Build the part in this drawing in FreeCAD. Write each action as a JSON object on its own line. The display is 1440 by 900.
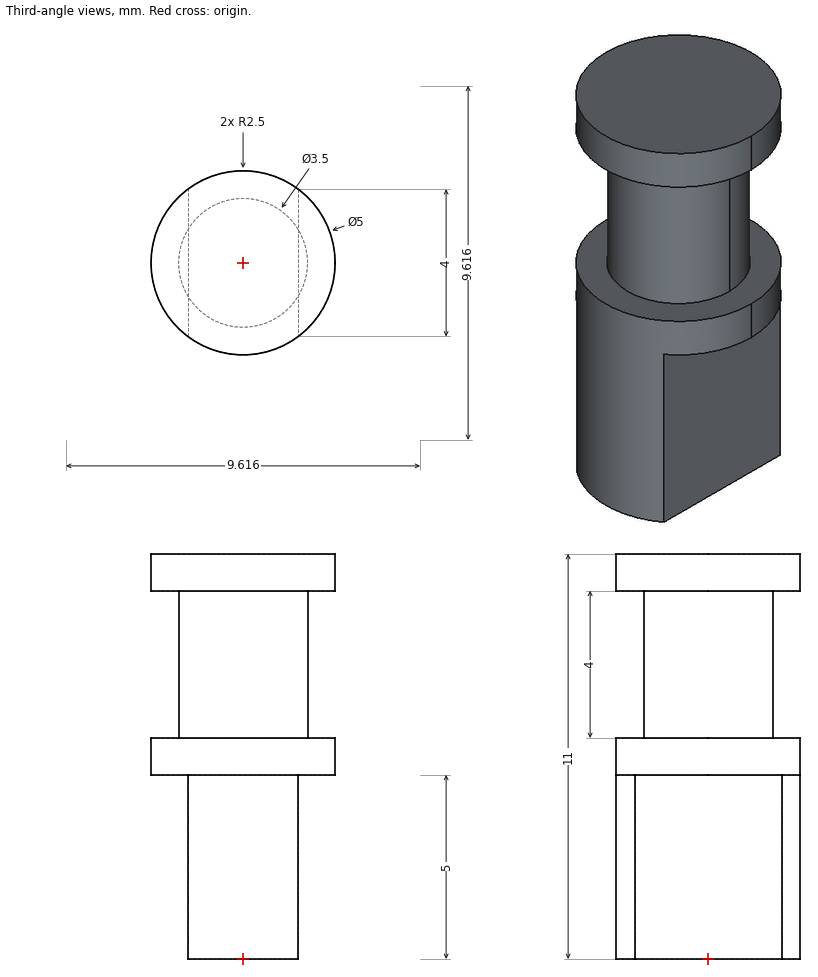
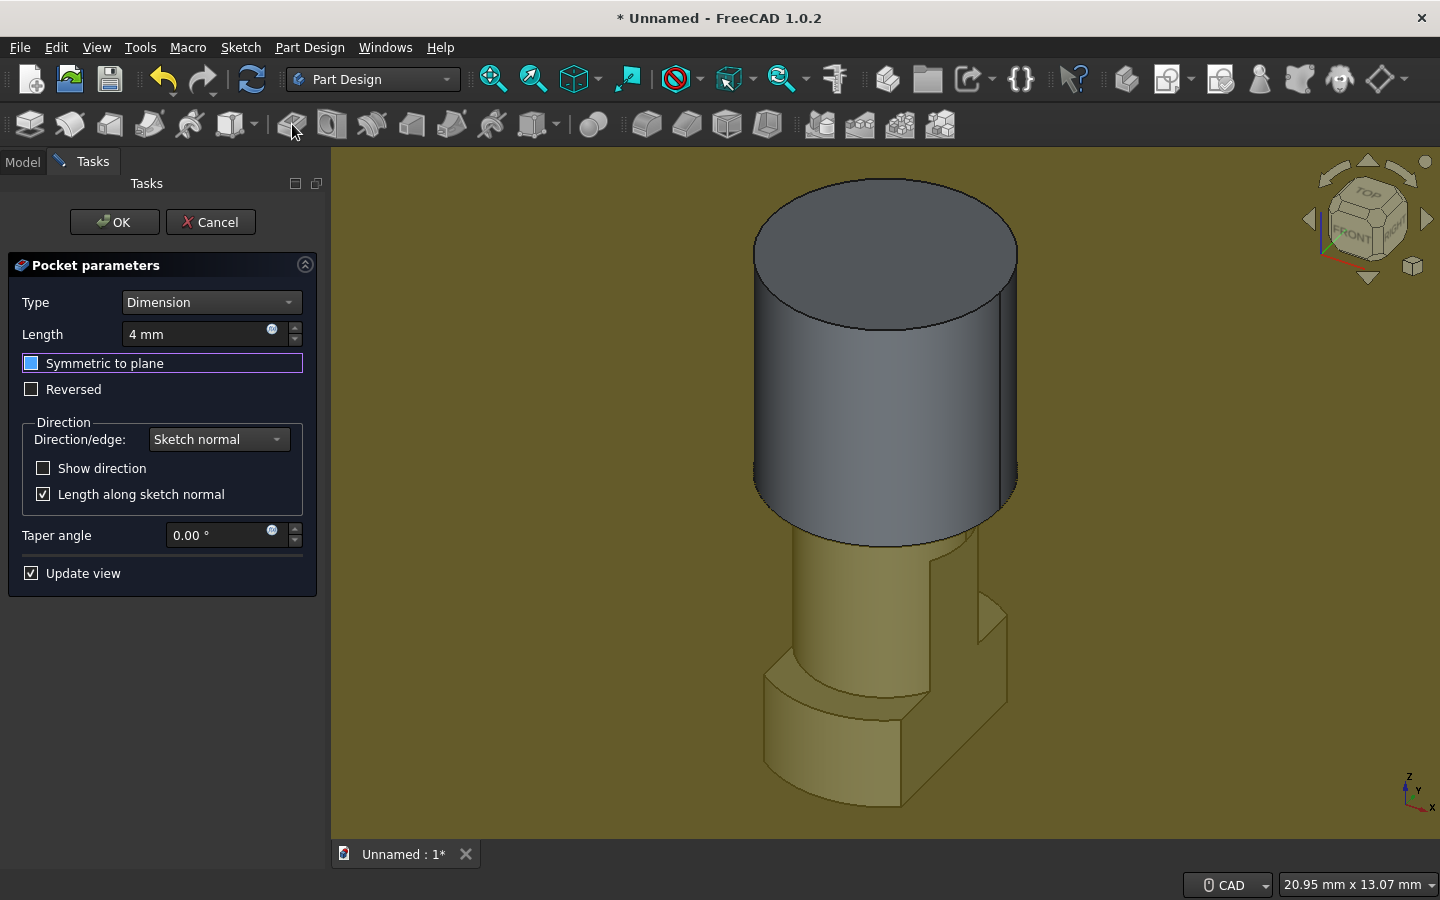
{"action": "left_click", "coordinate": [30, 389]}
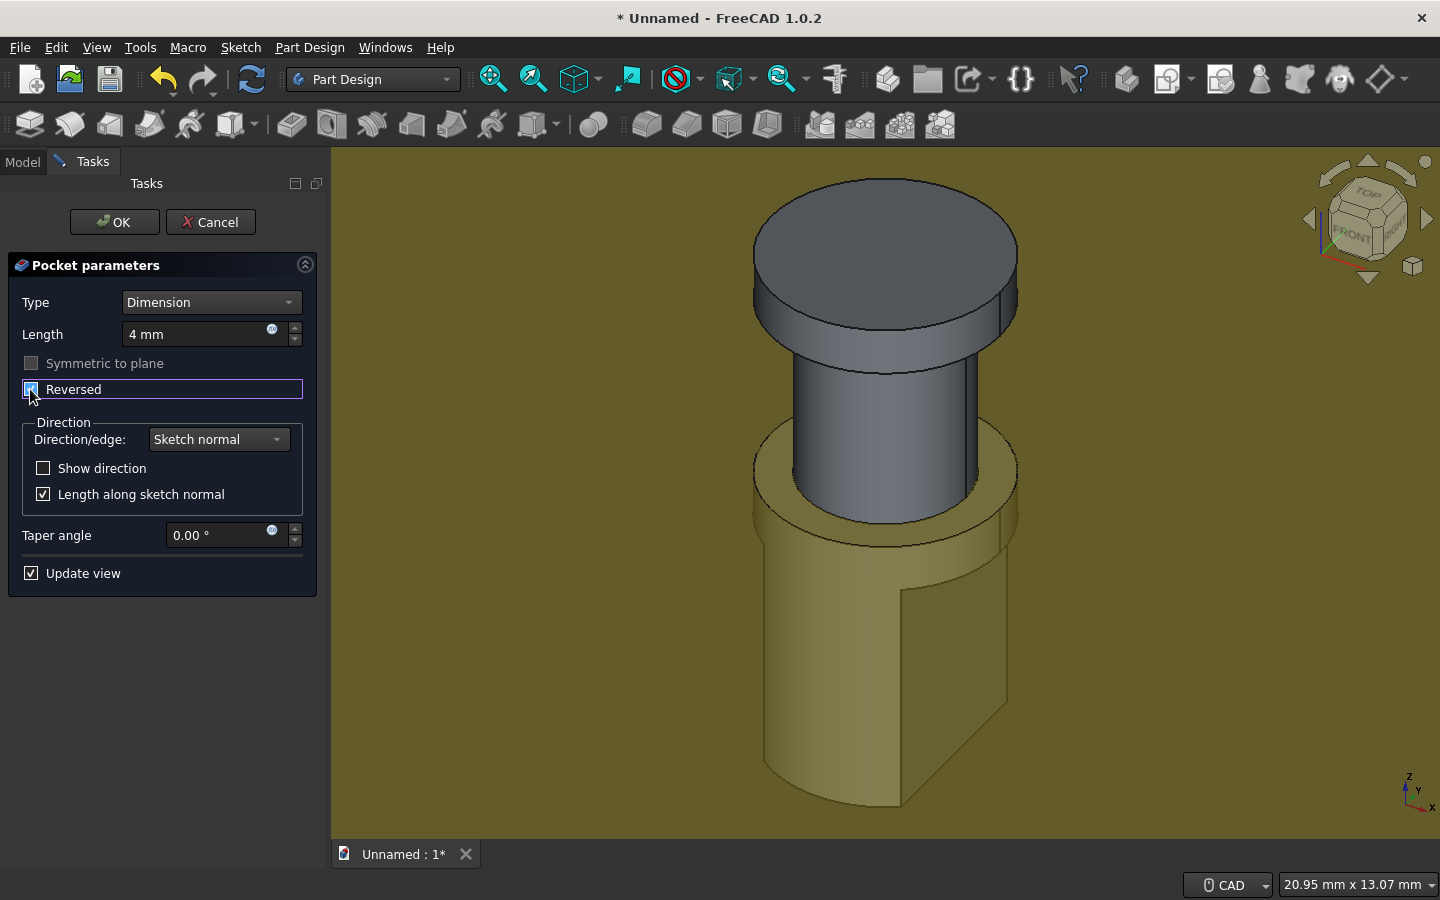
{"action": "left_click", "coordinate": [115, 222]}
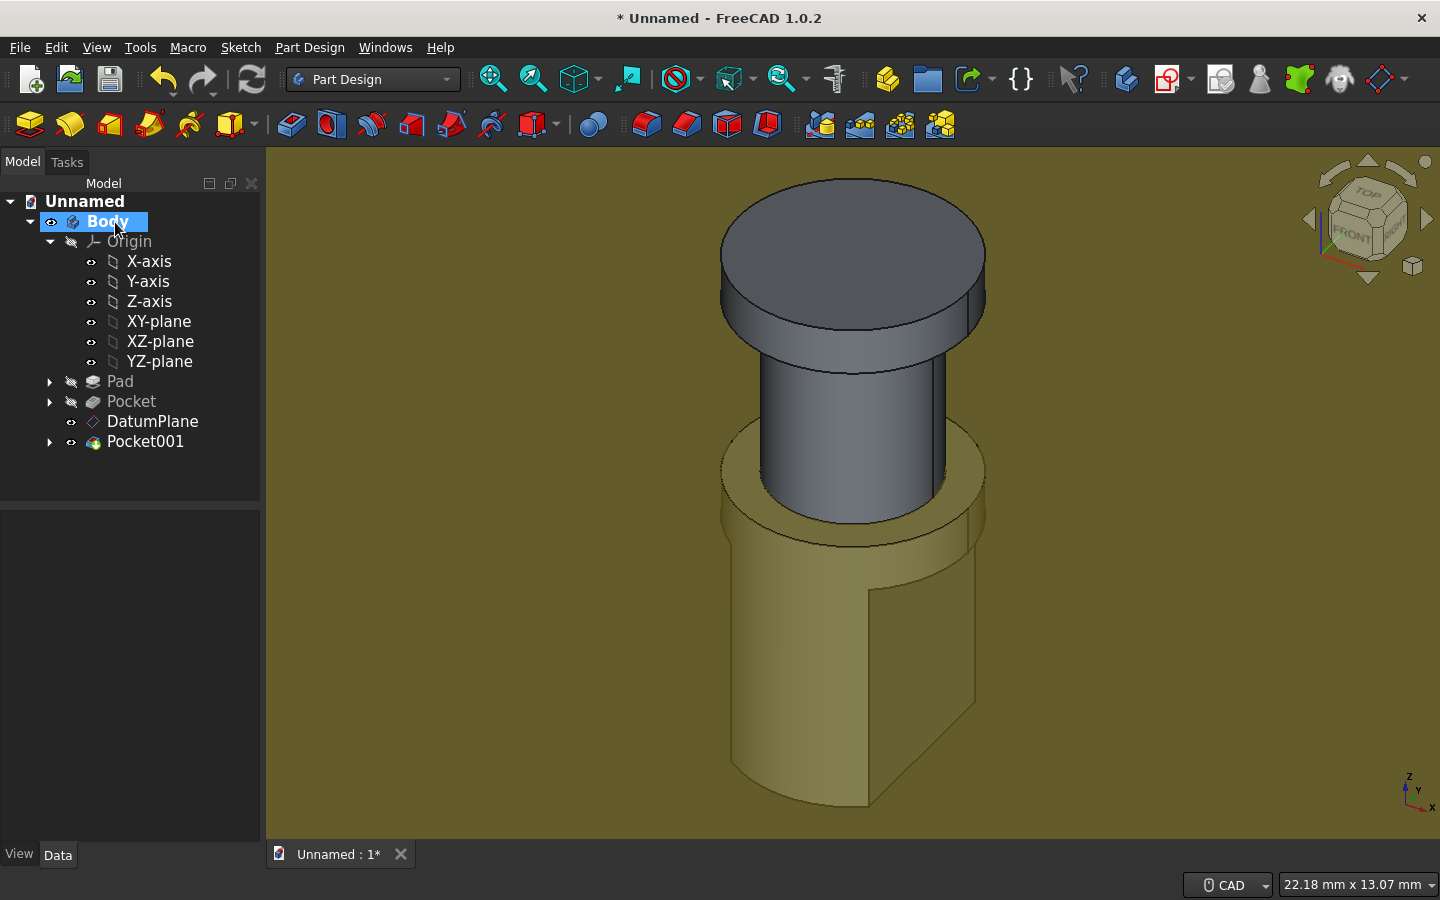
{"action": "left_click", "coordinate": [116, 422]}
{"action": "key", "text": "space"}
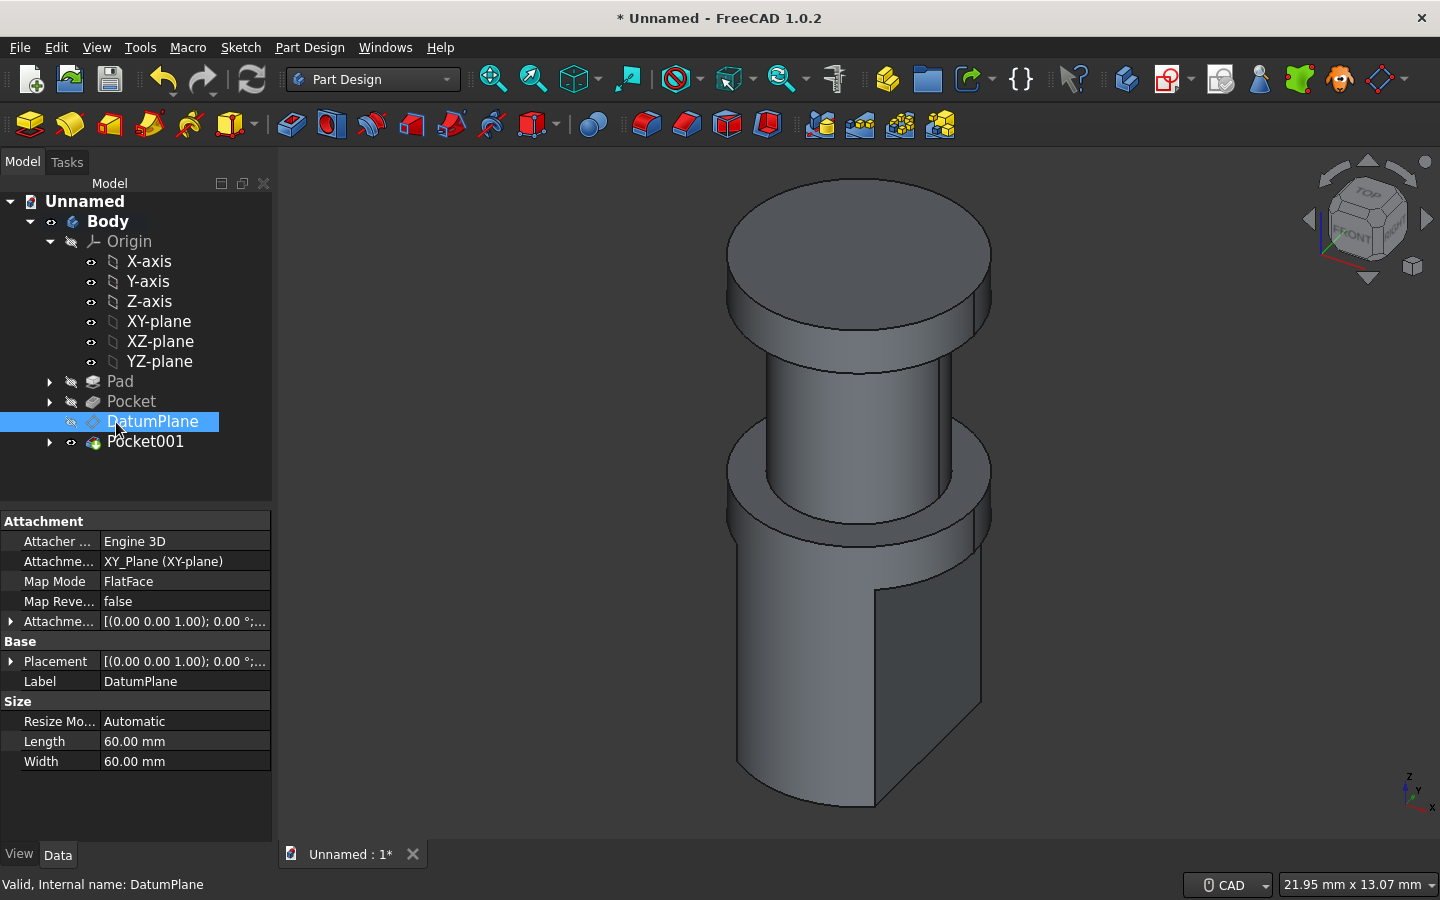
{"action": "key", "text": "0"}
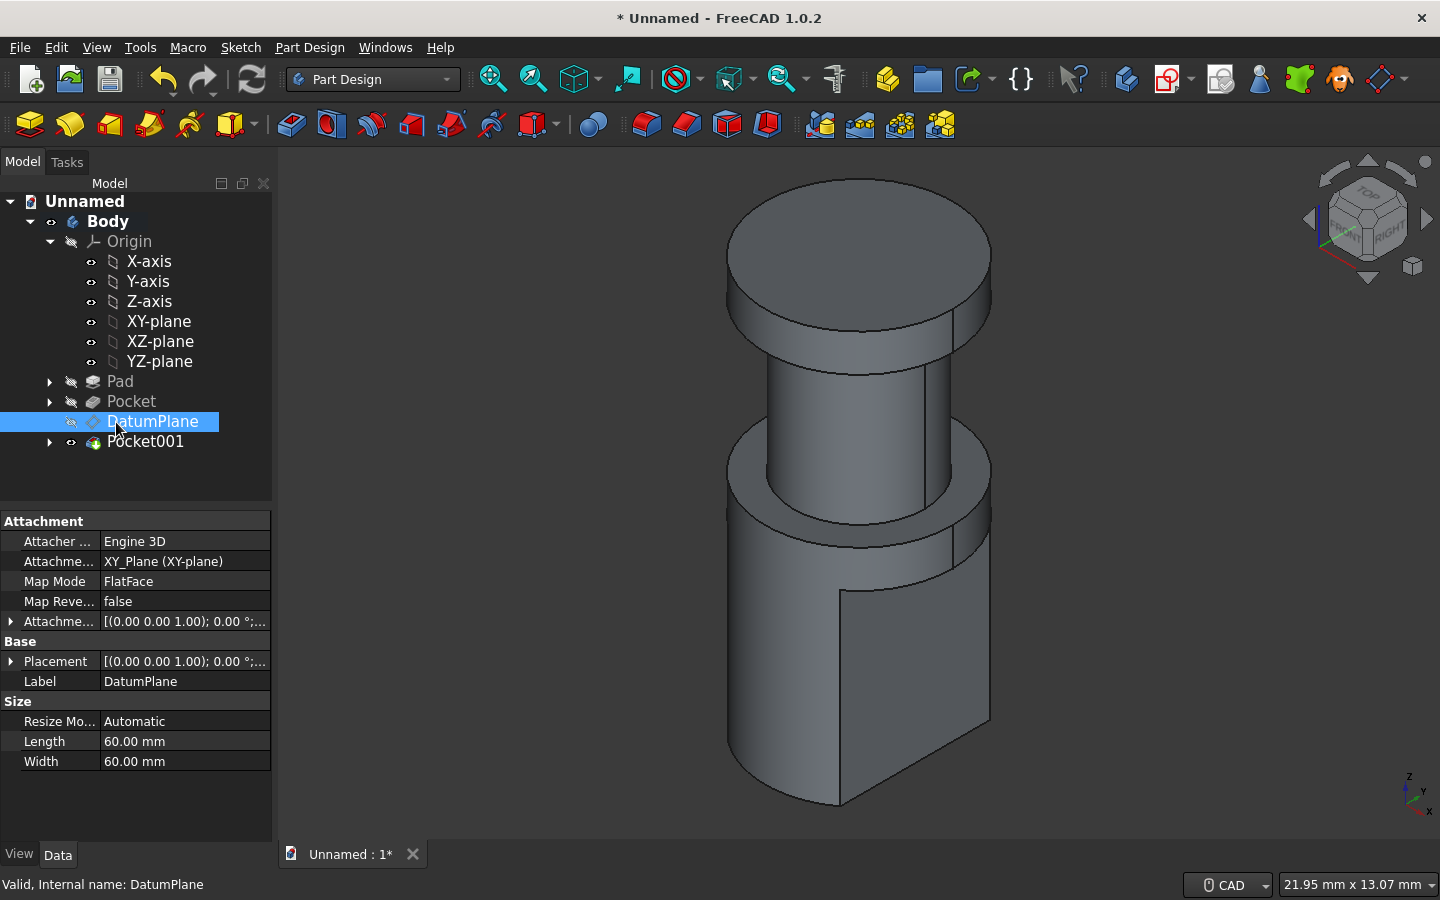
{"action": "left_click", "coordinate": [494, 80]}